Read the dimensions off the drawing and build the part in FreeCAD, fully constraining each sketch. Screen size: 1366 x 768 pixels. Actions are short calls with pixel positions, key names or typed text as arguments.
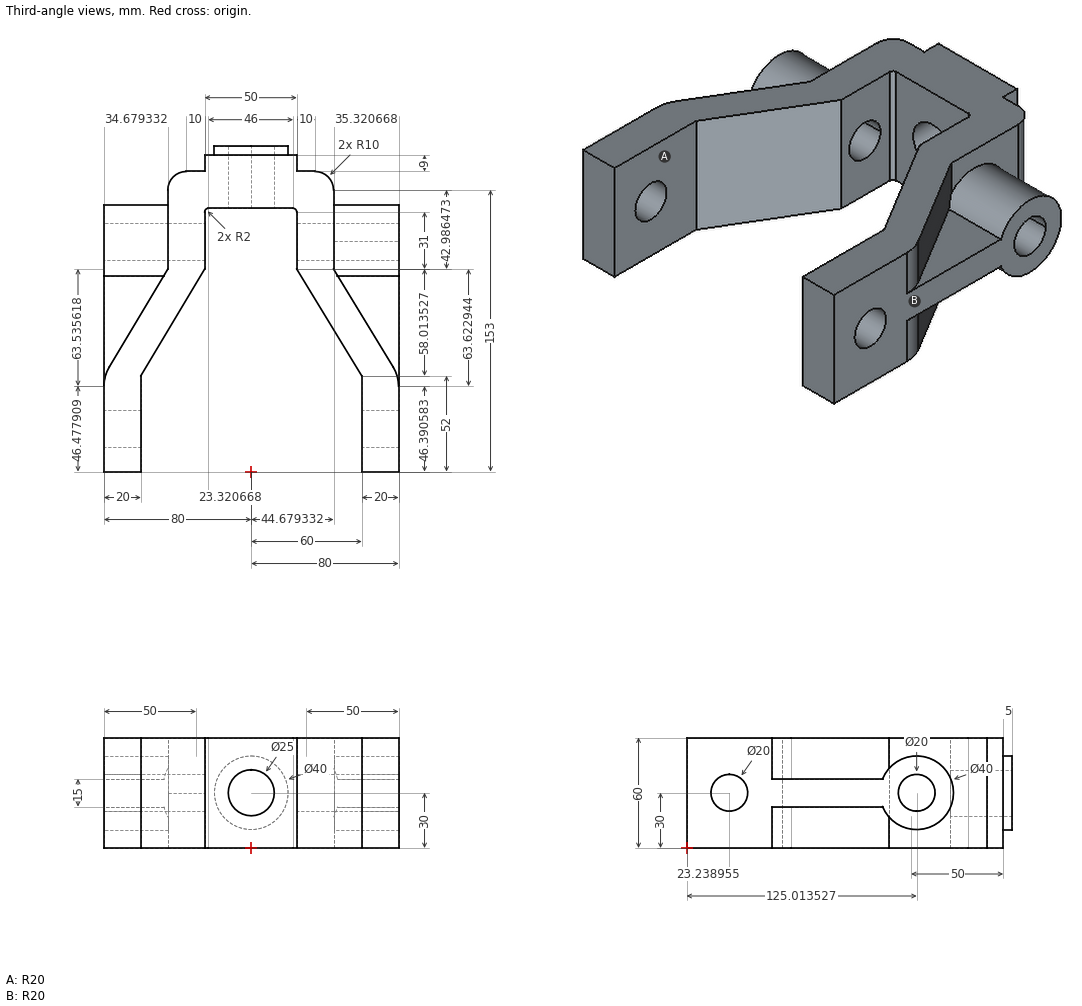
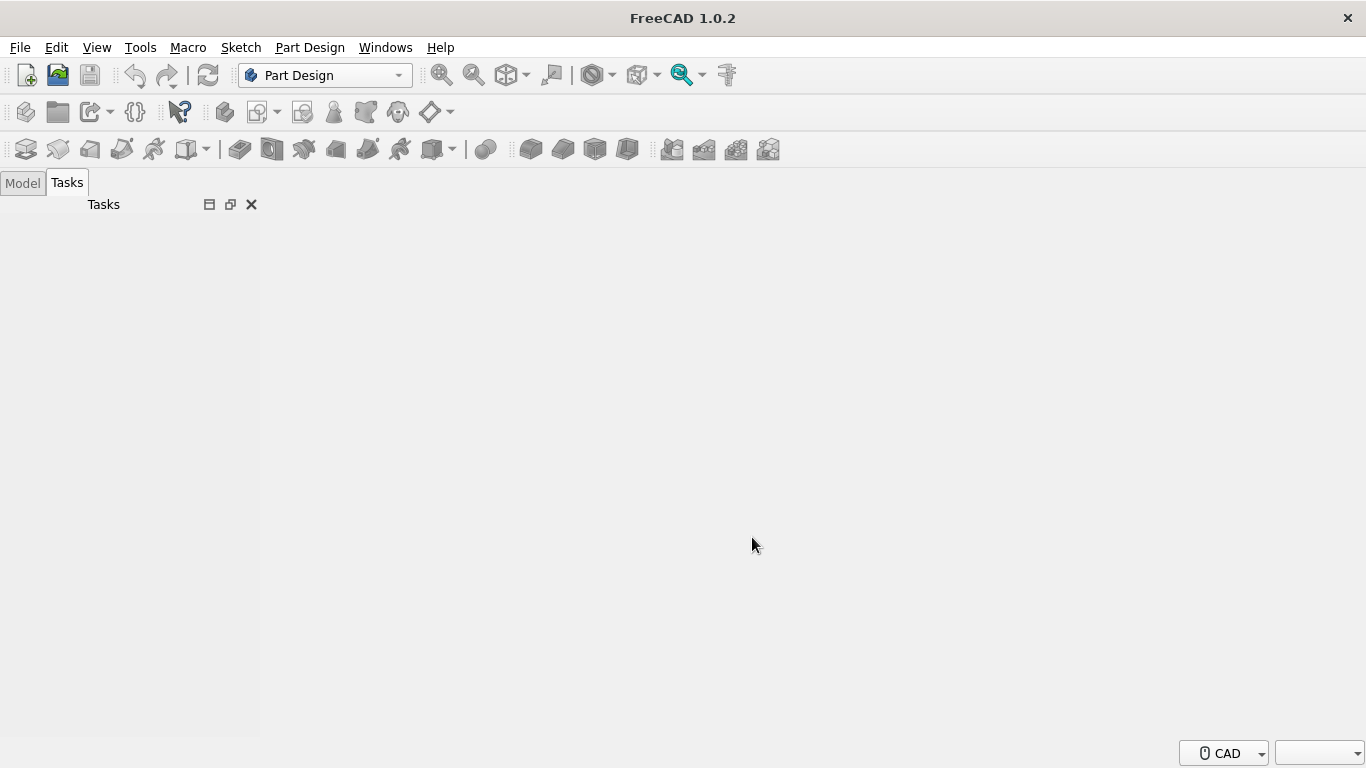
click(26, 76)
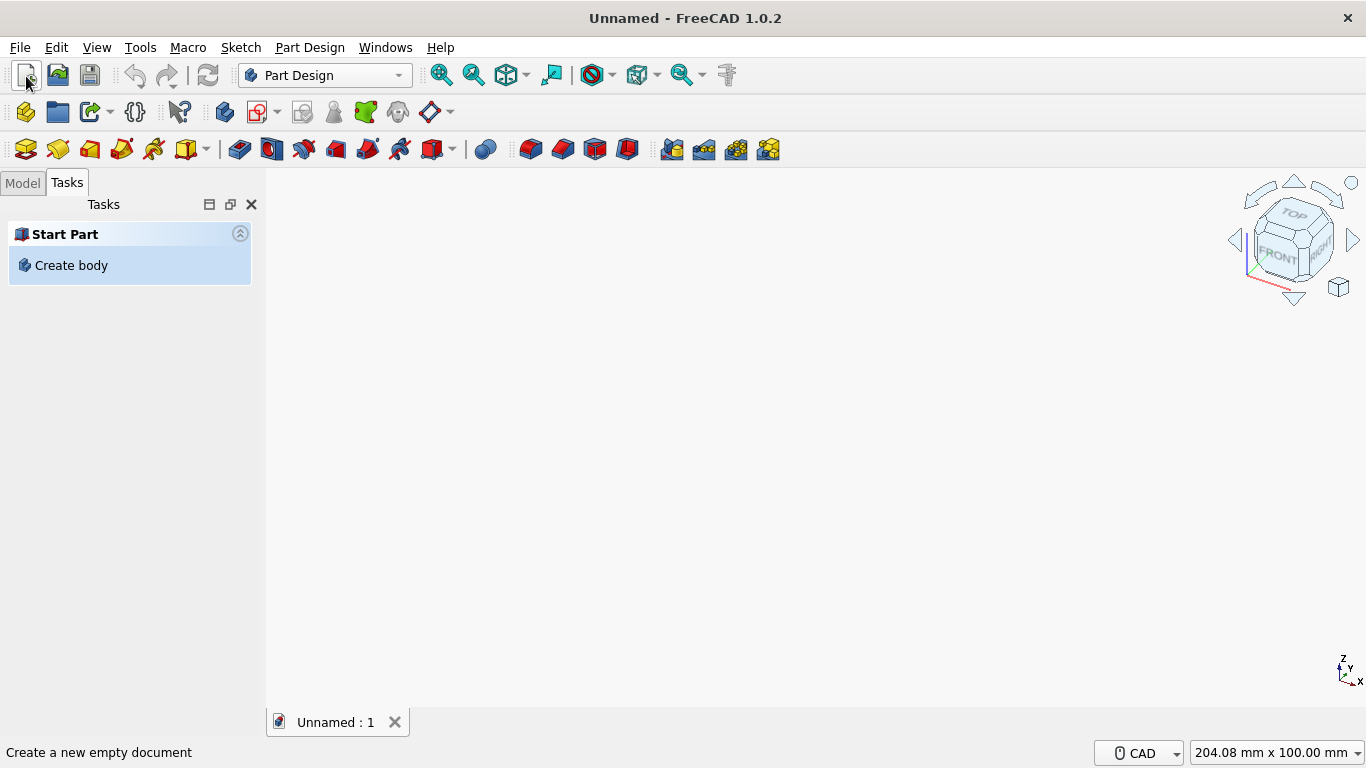
click(258, 112)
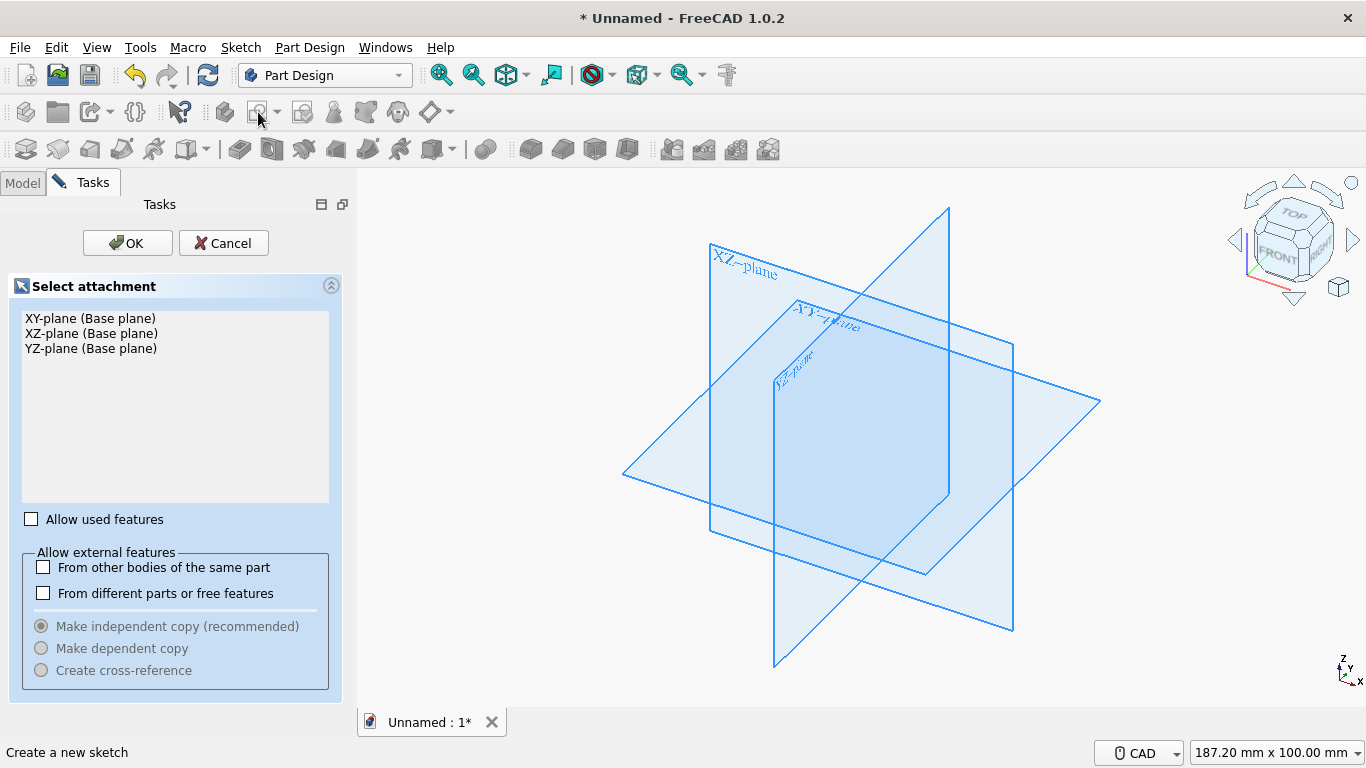
click(82, 318)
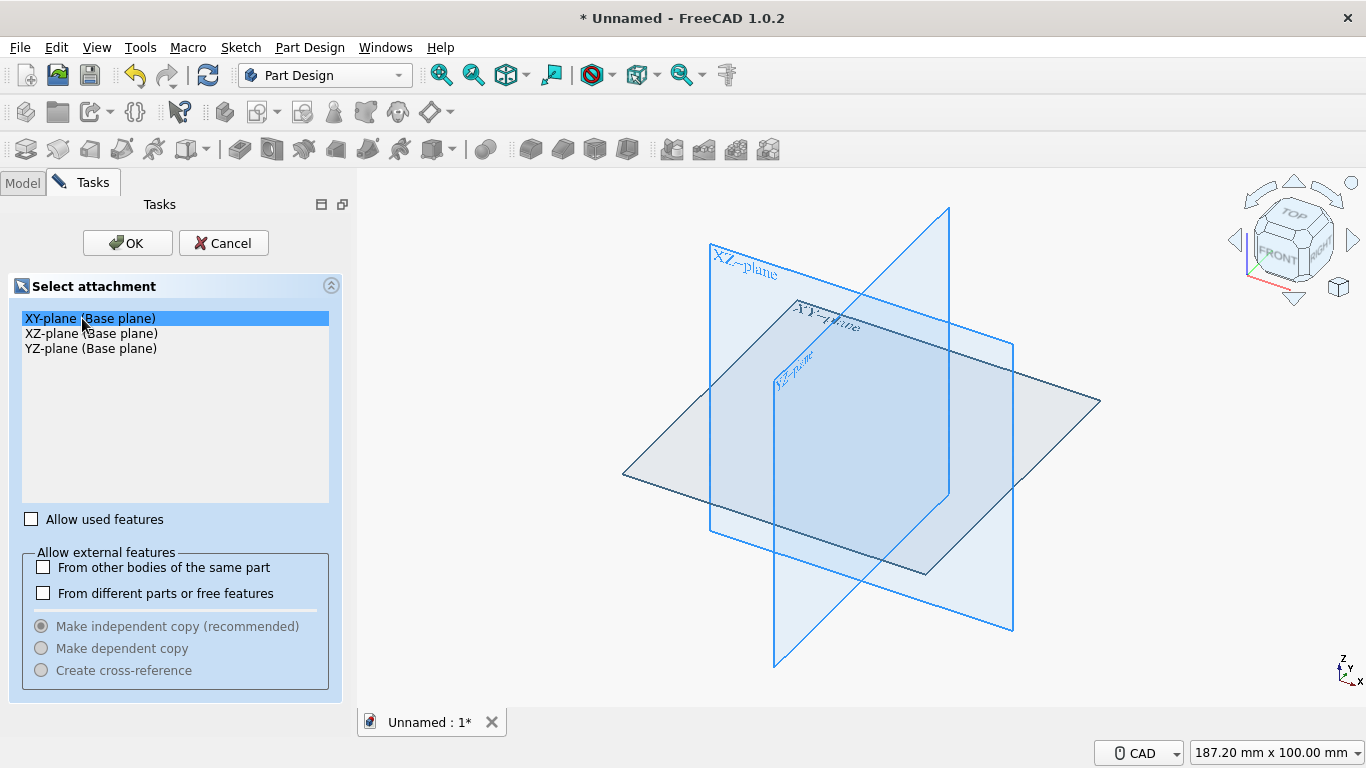
click(128, 243)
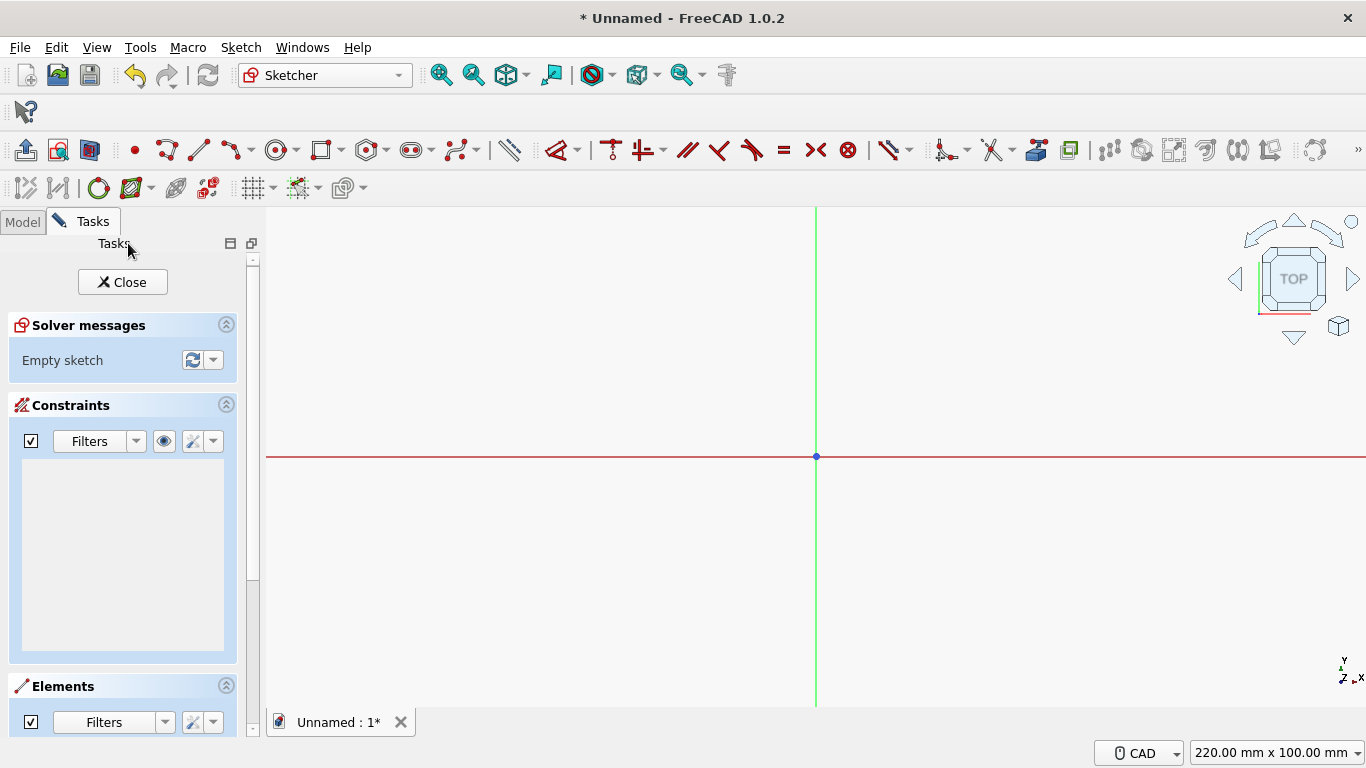
scroll(708, 679, down, 5)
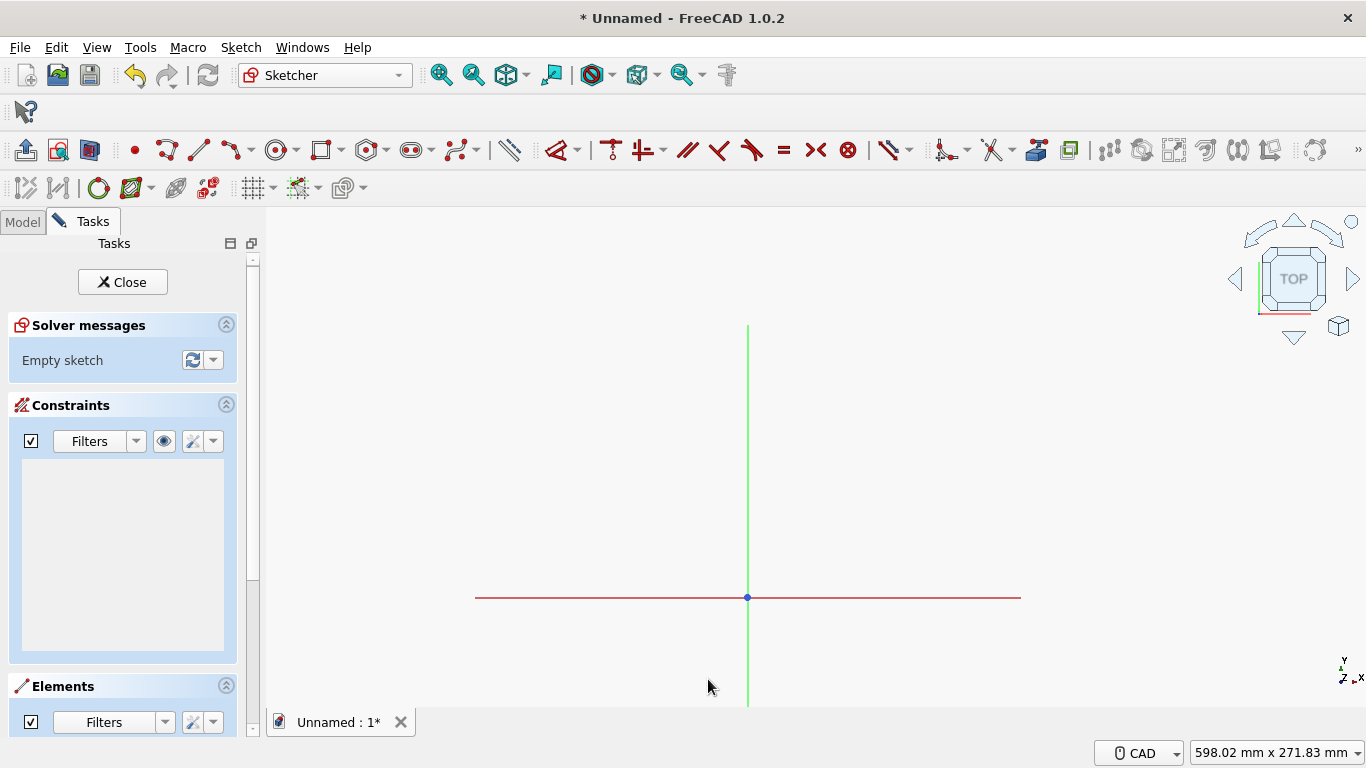
key(g)
key(l)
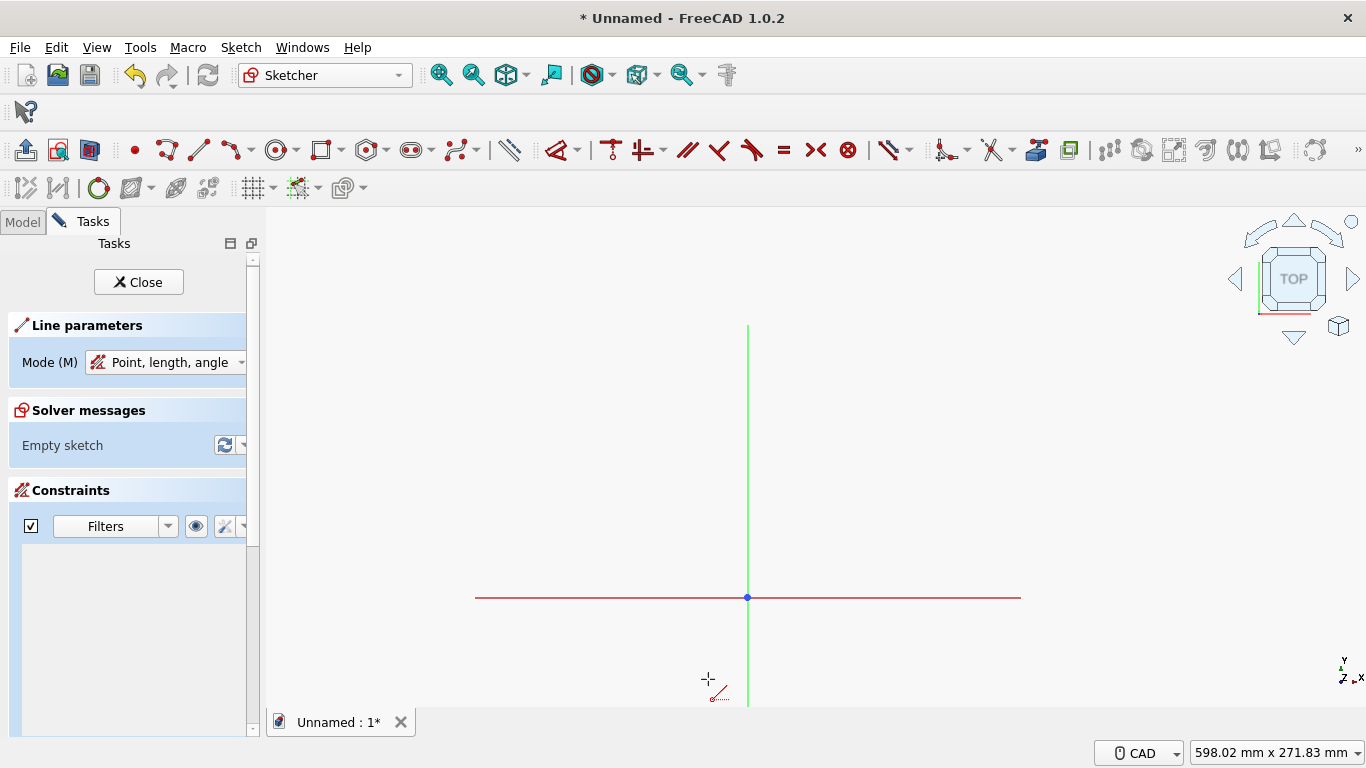
click(705, 335)
click(790, 335)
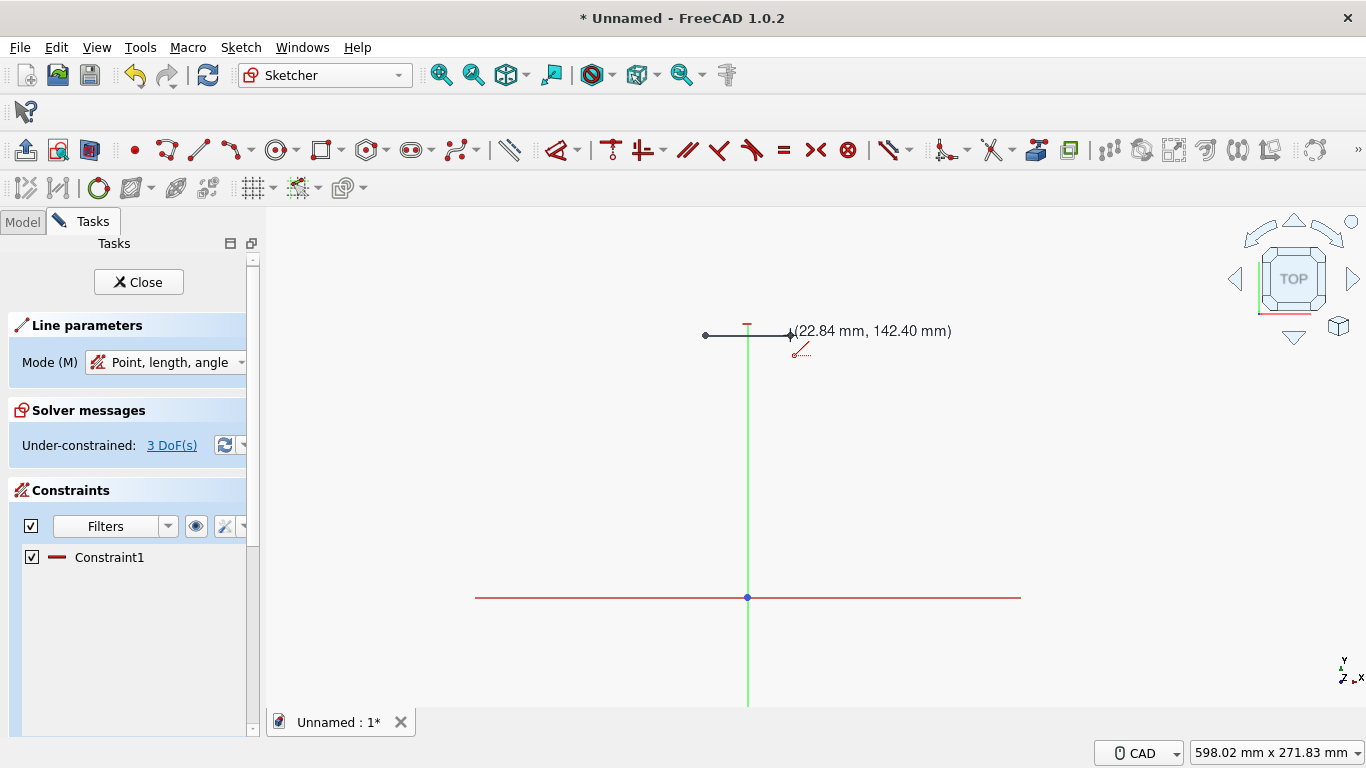
key(g)
key(m)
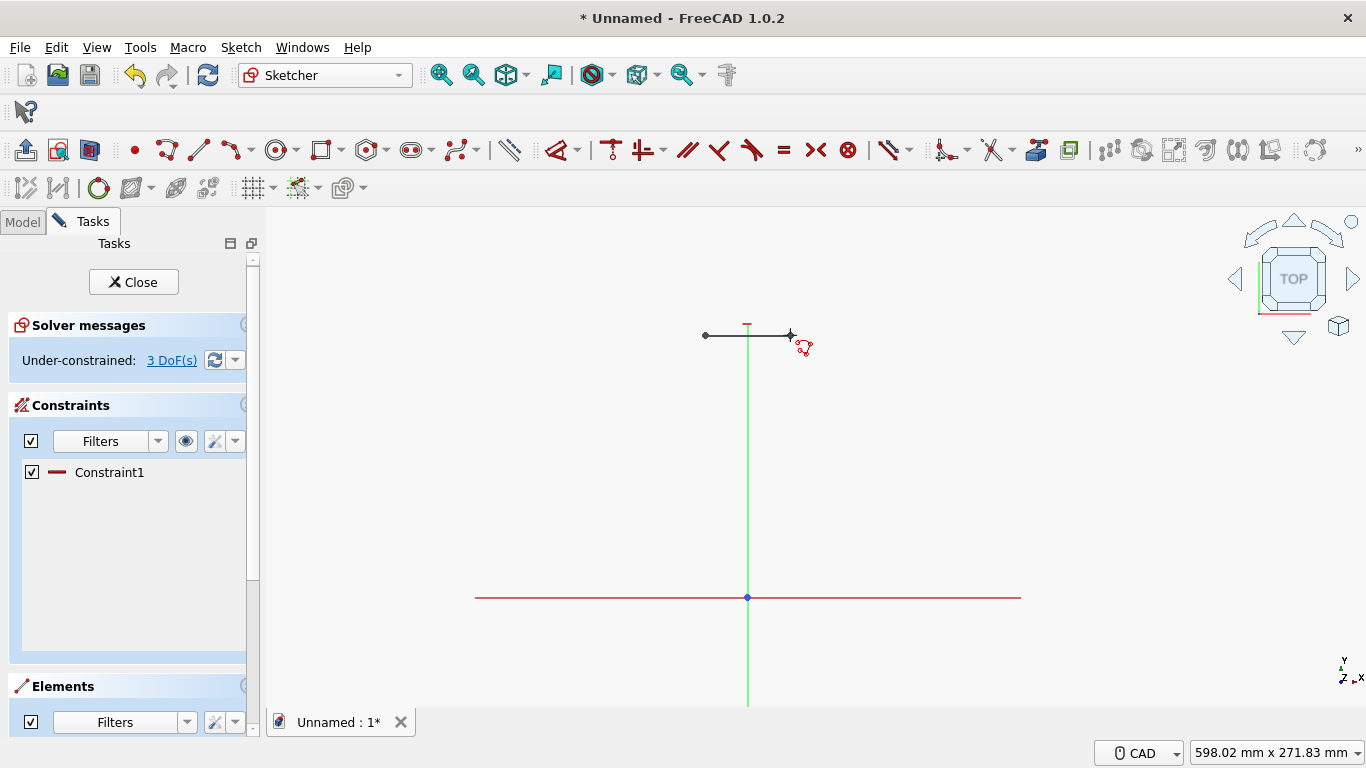
scroll(793, 339, up, 6)